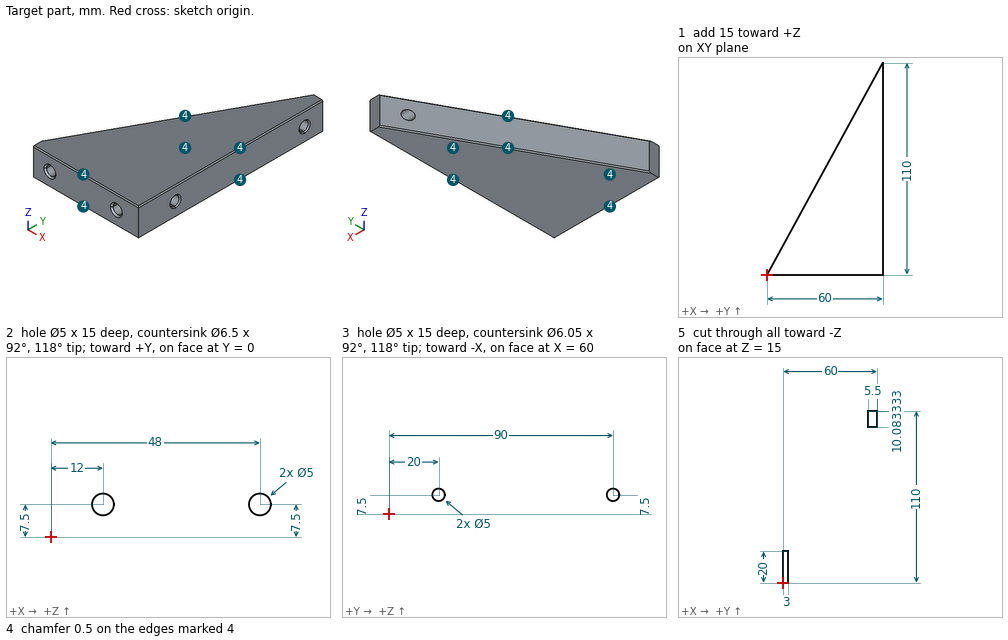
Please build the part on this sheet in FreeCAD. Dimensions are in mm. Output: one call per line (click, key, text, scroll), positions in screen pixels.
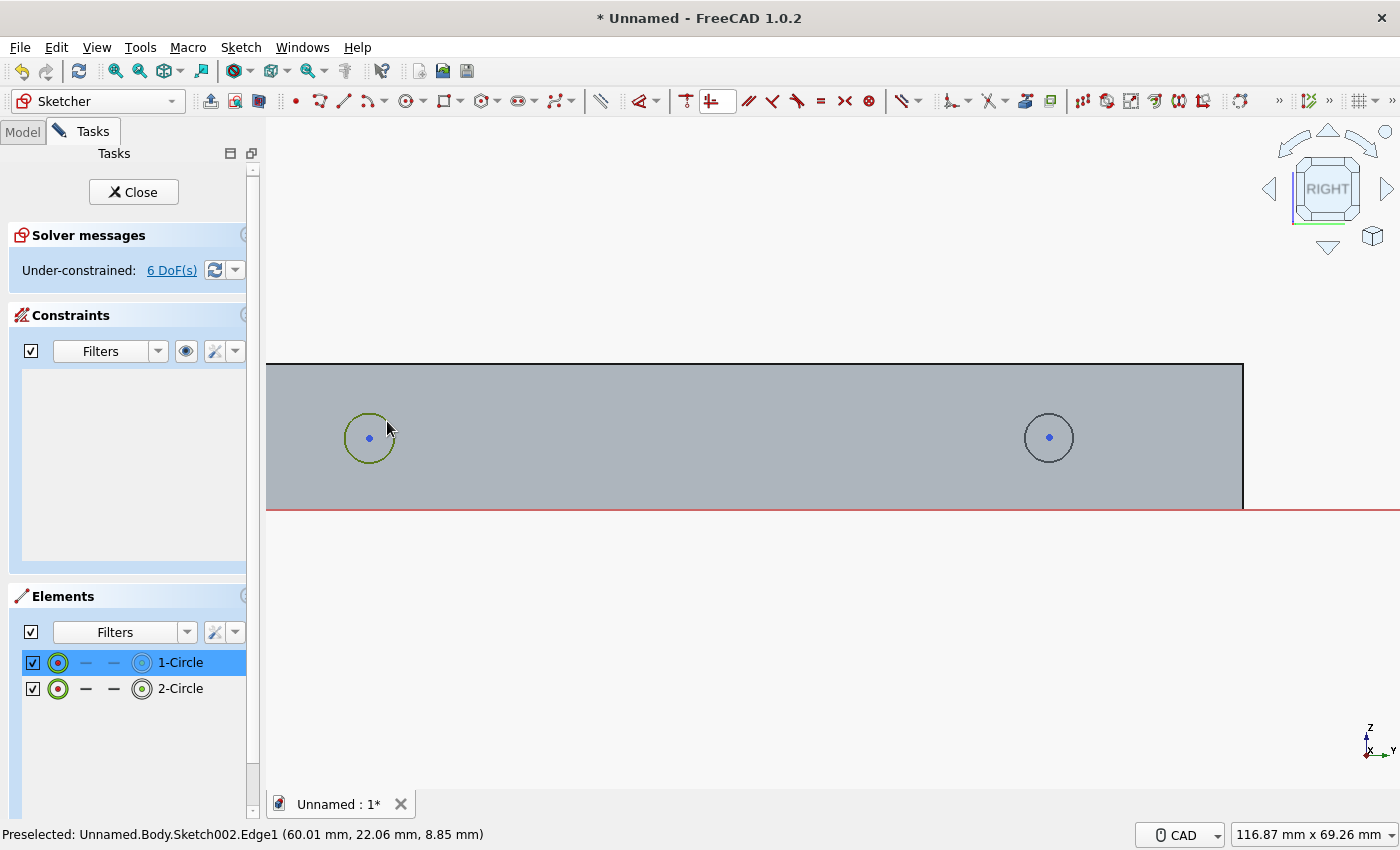
click(1066, 421)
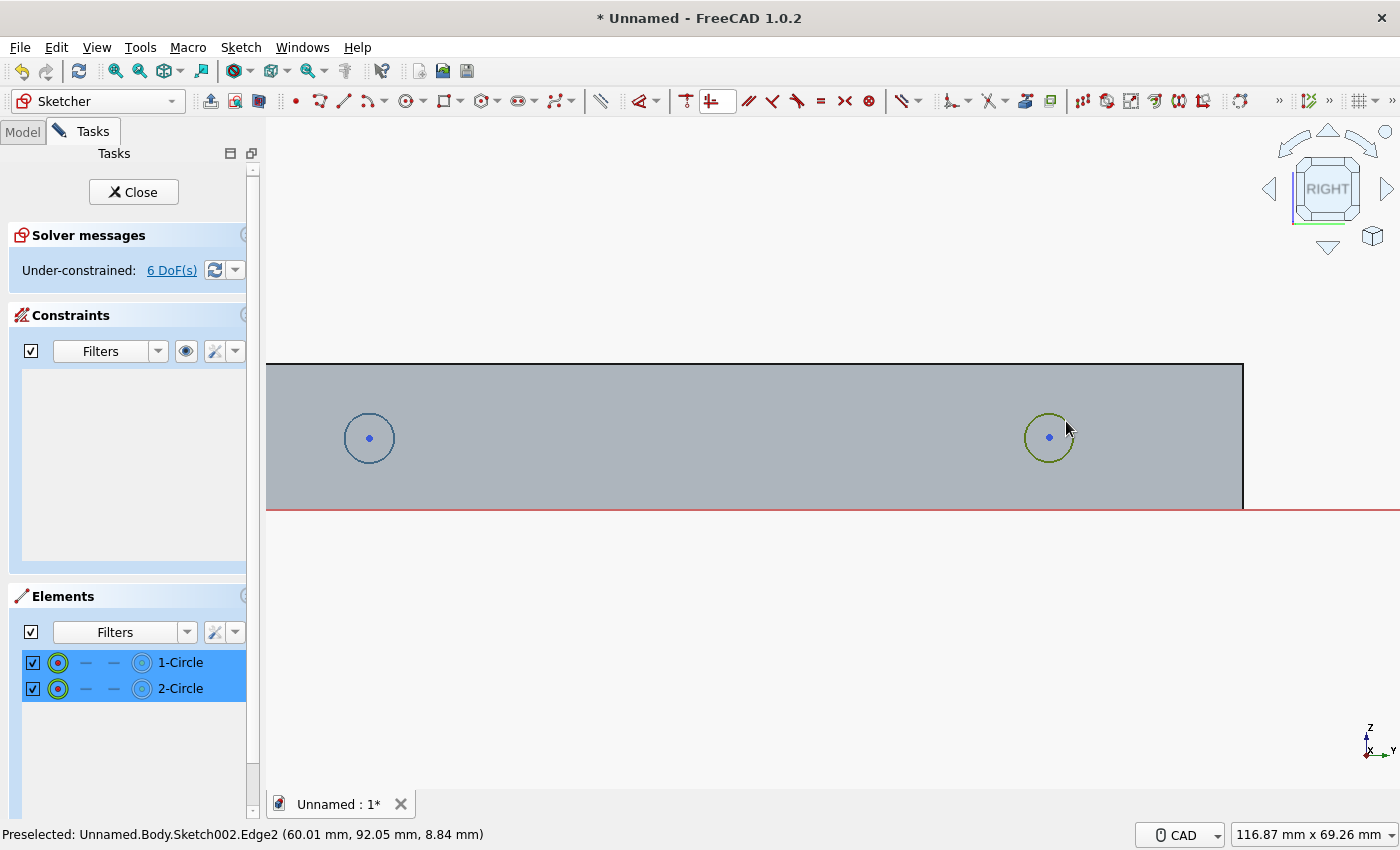
click(822, 102)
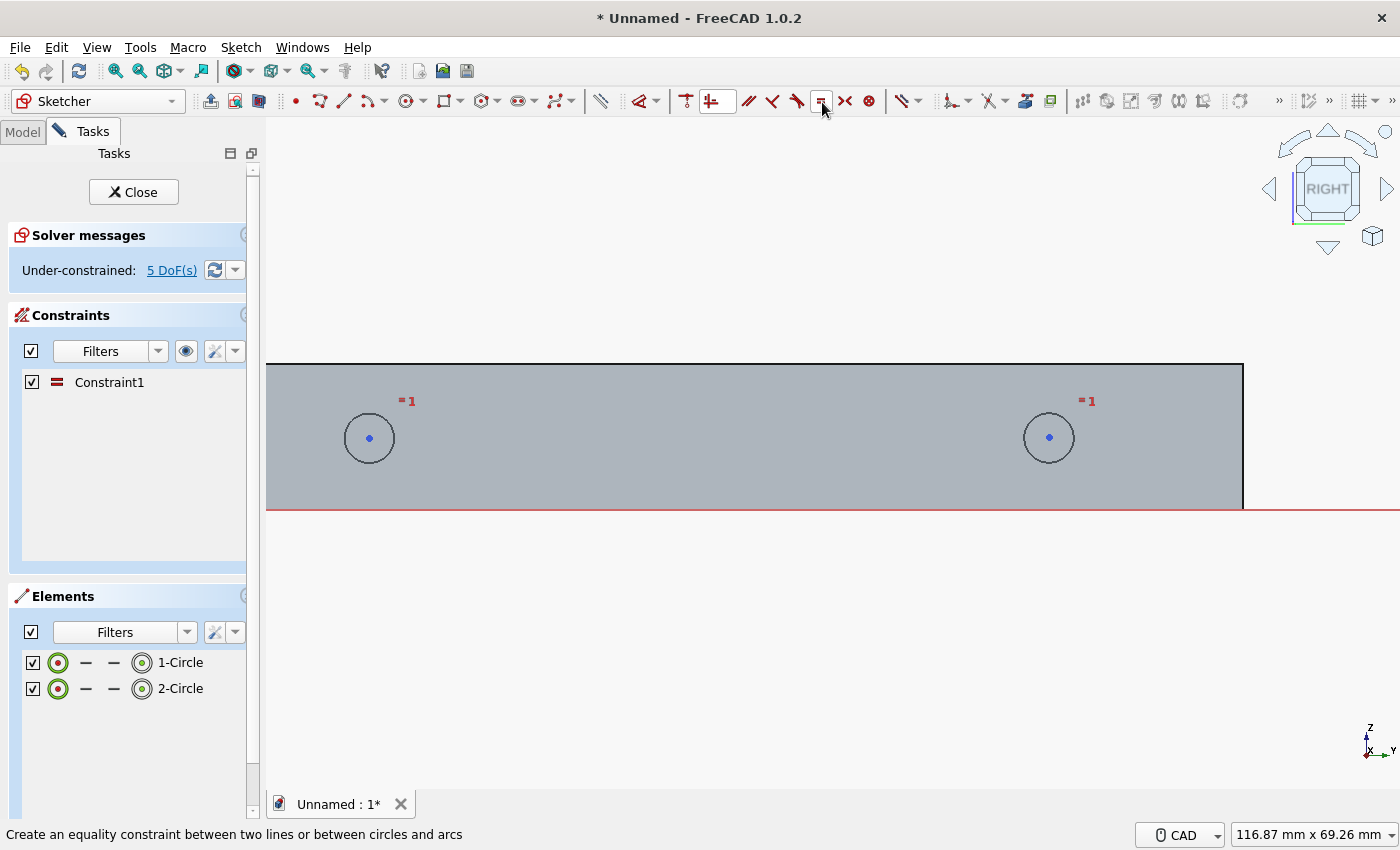
click(640, 102)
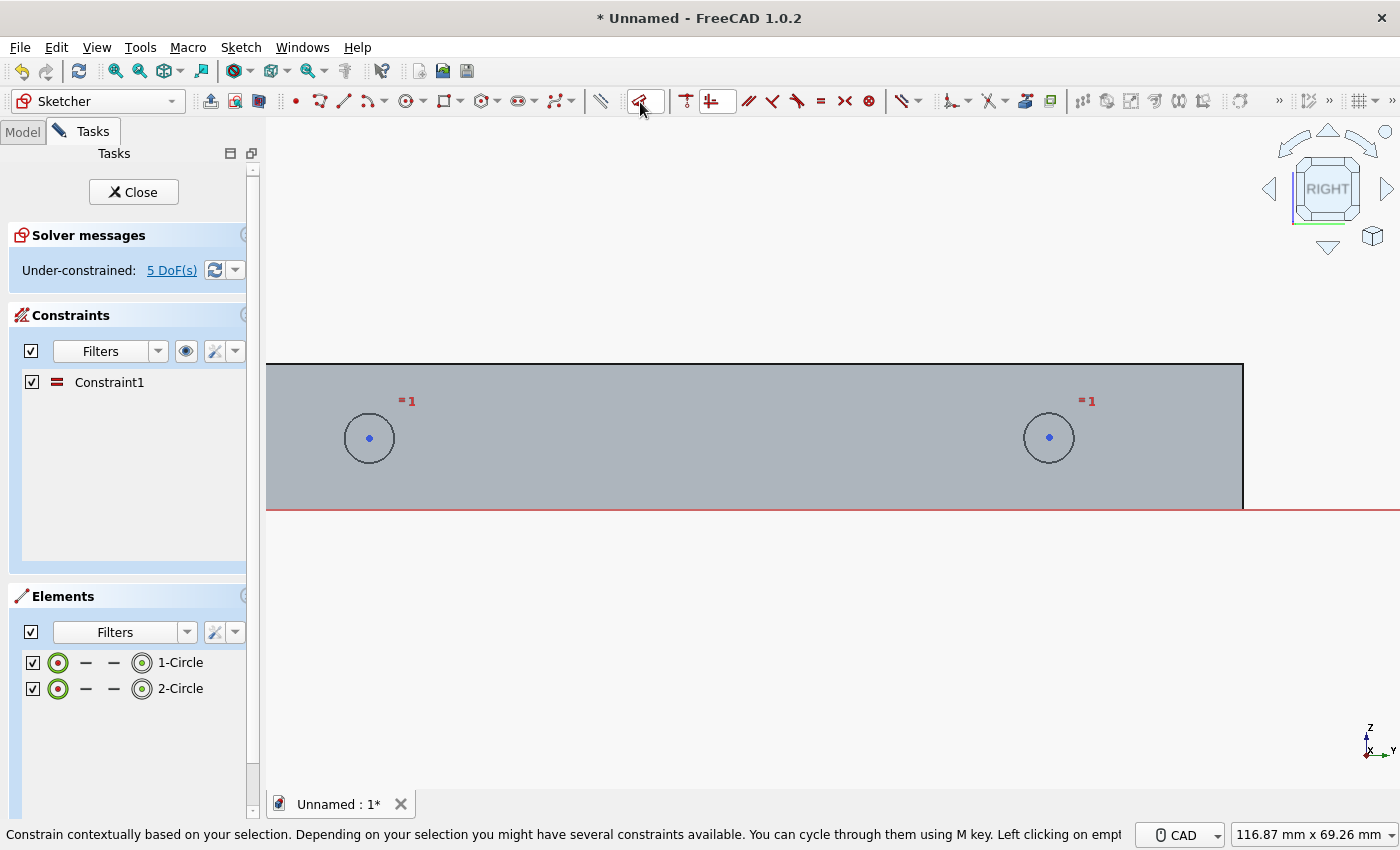
click(387, 421)
click(410, 399)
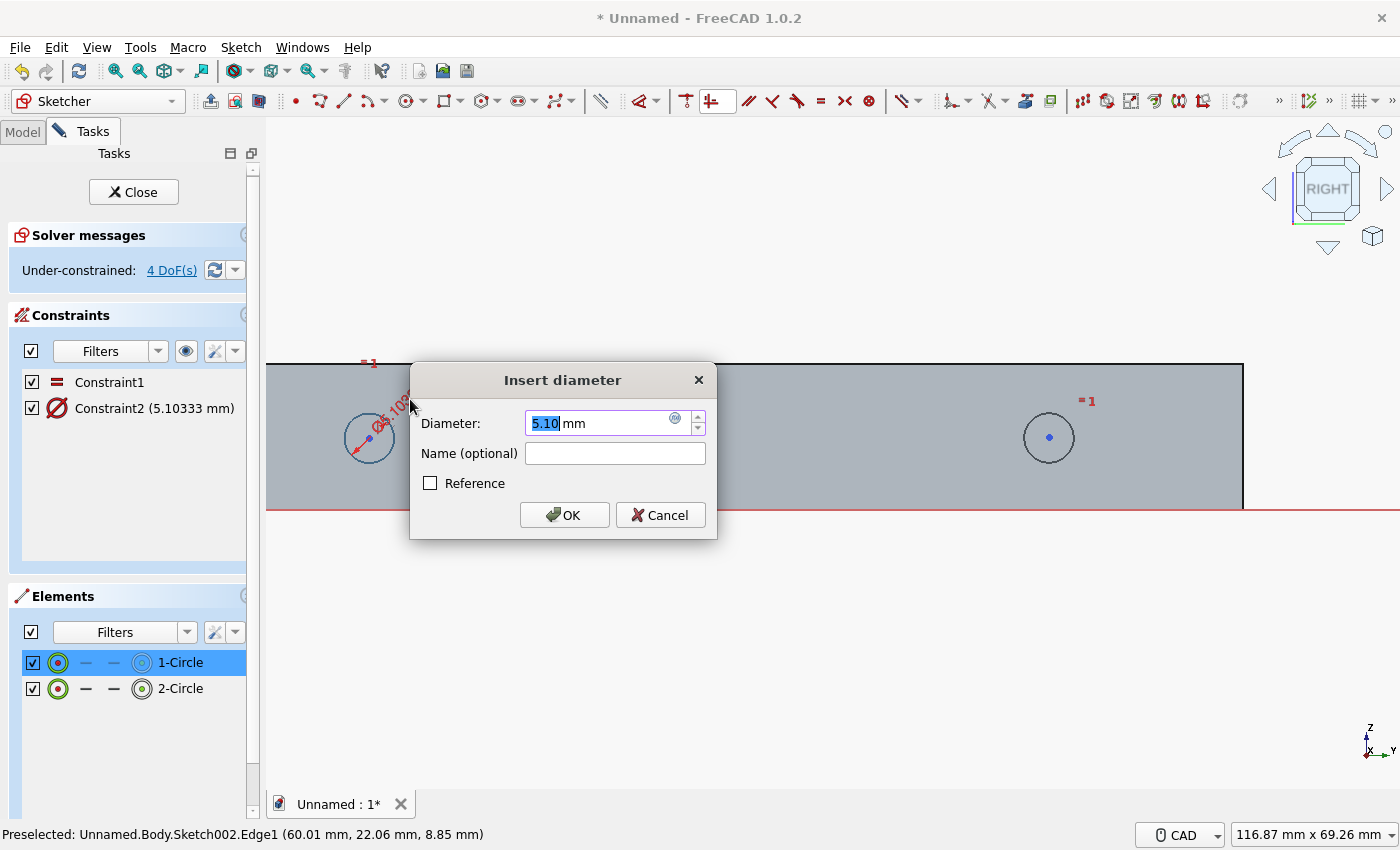
text(5)
key(Return)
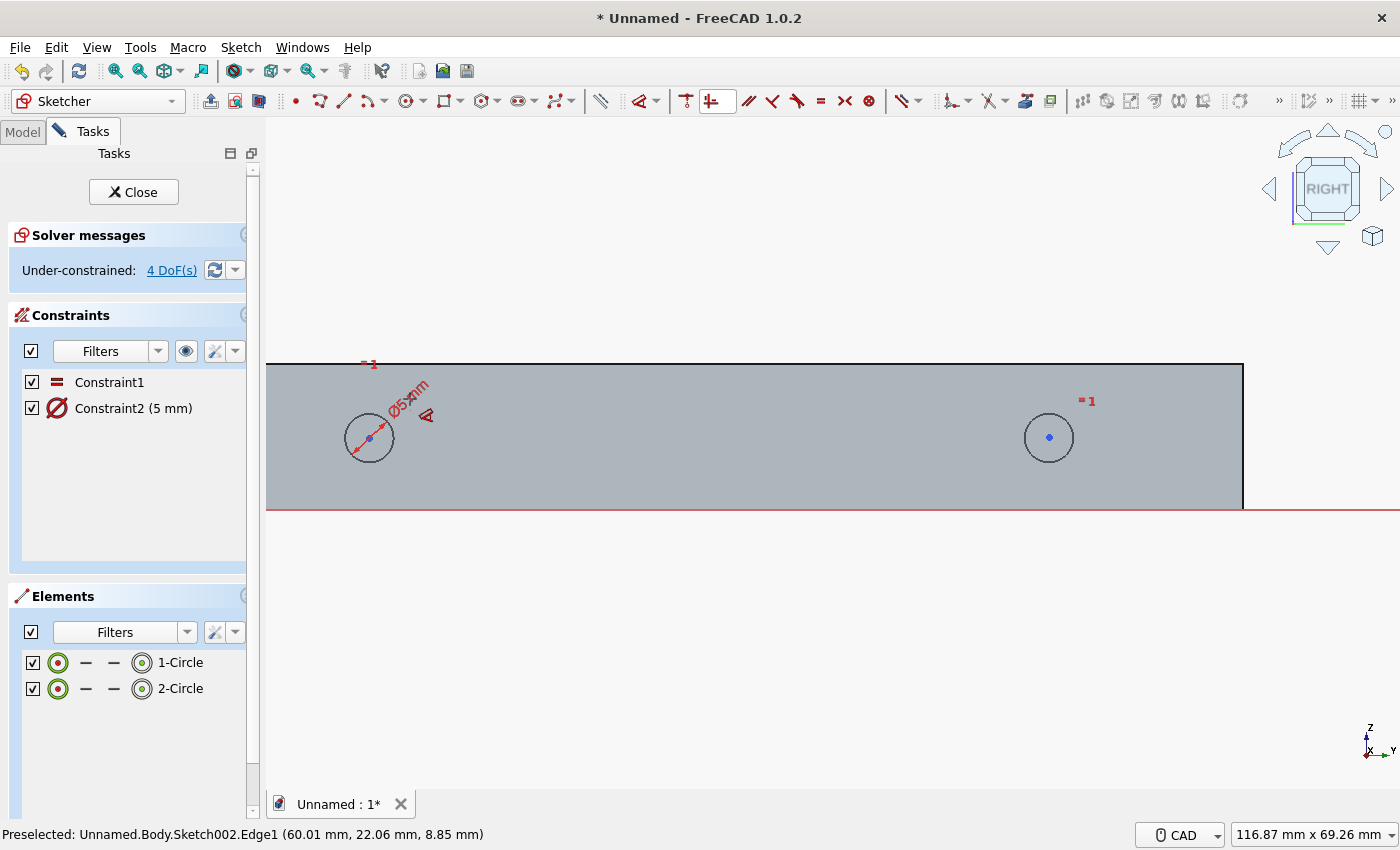
click(369, 438)
click(332, 544)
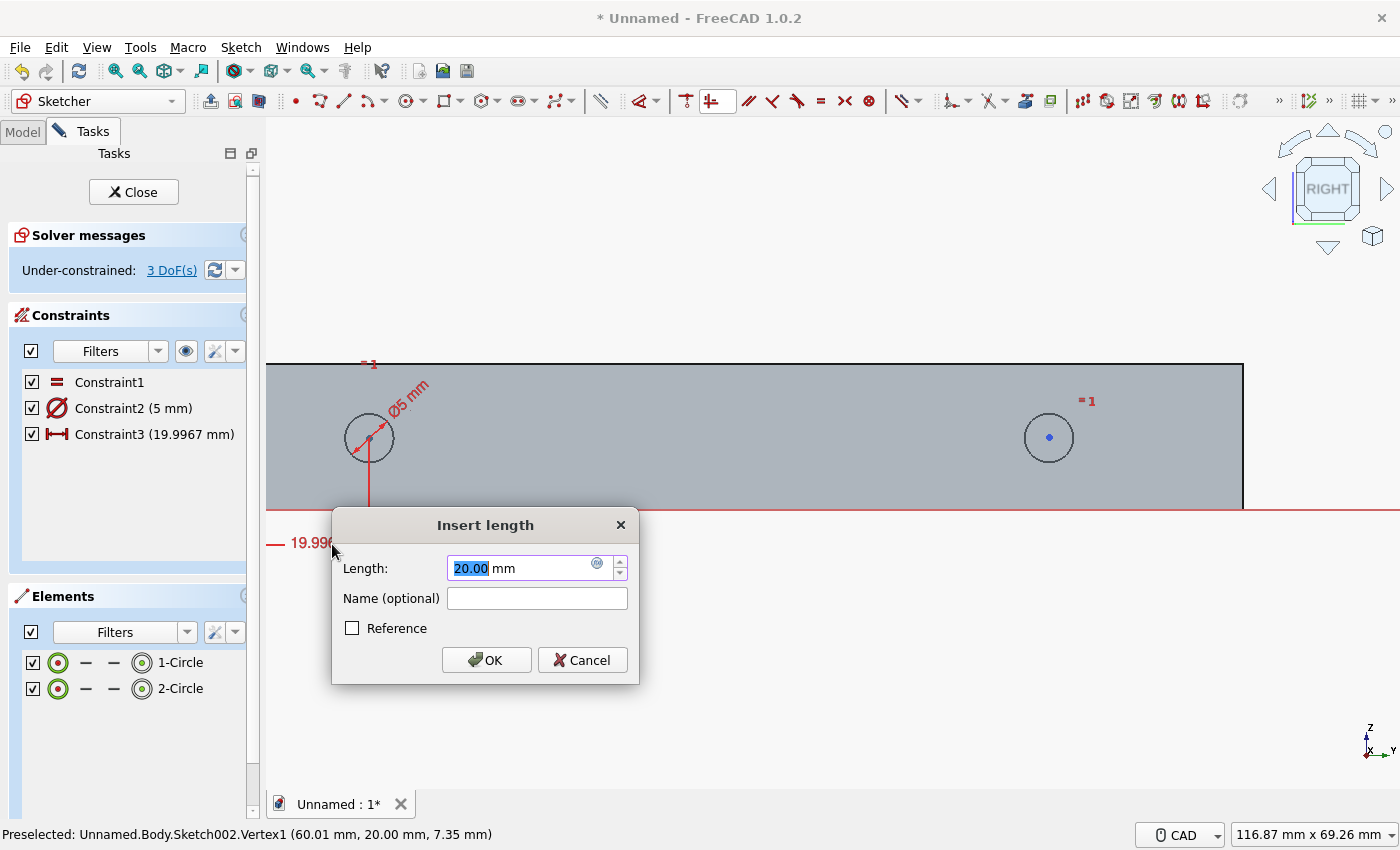
text(20)
key(Return)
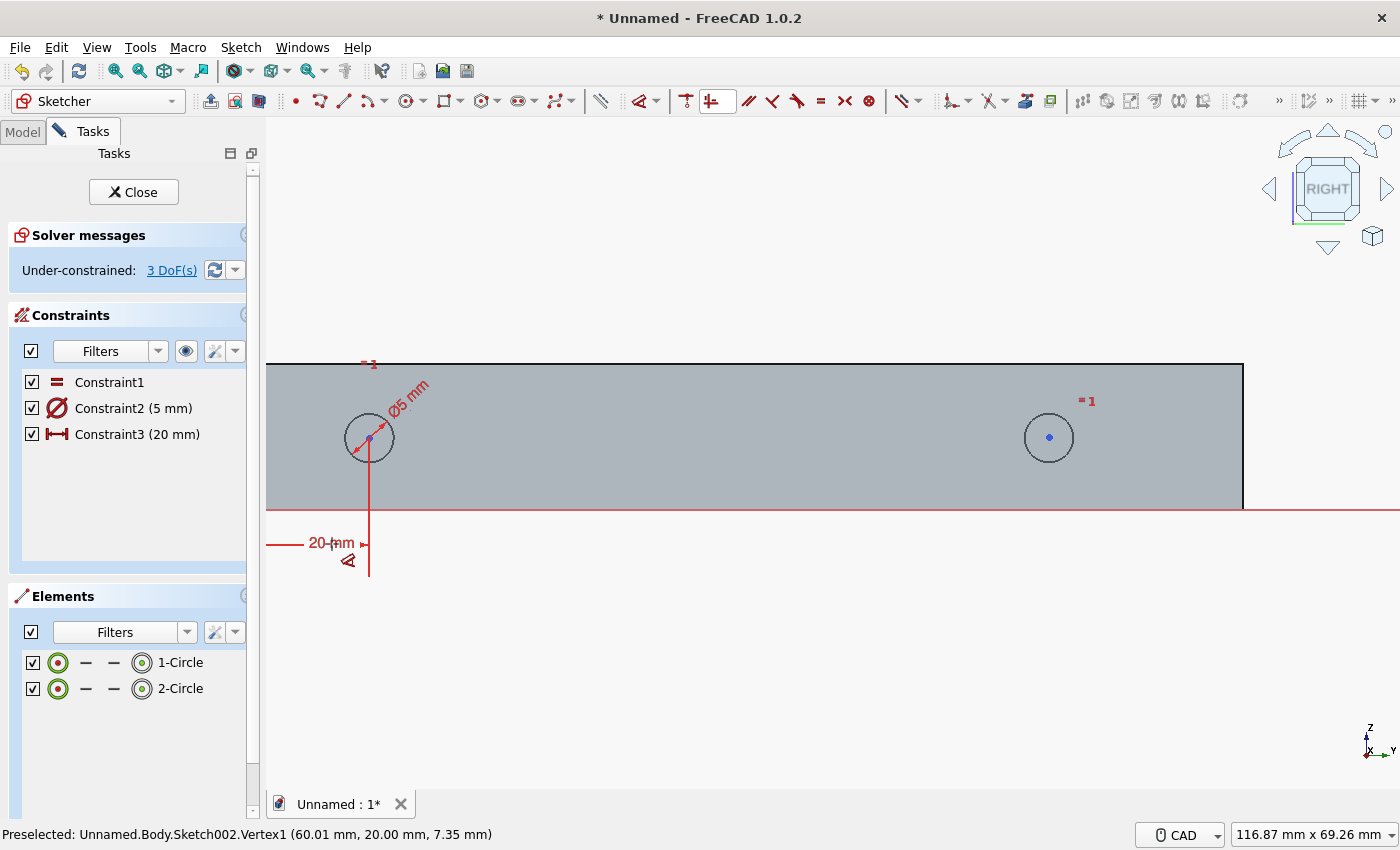
click(1049, 438)
click(671, 544)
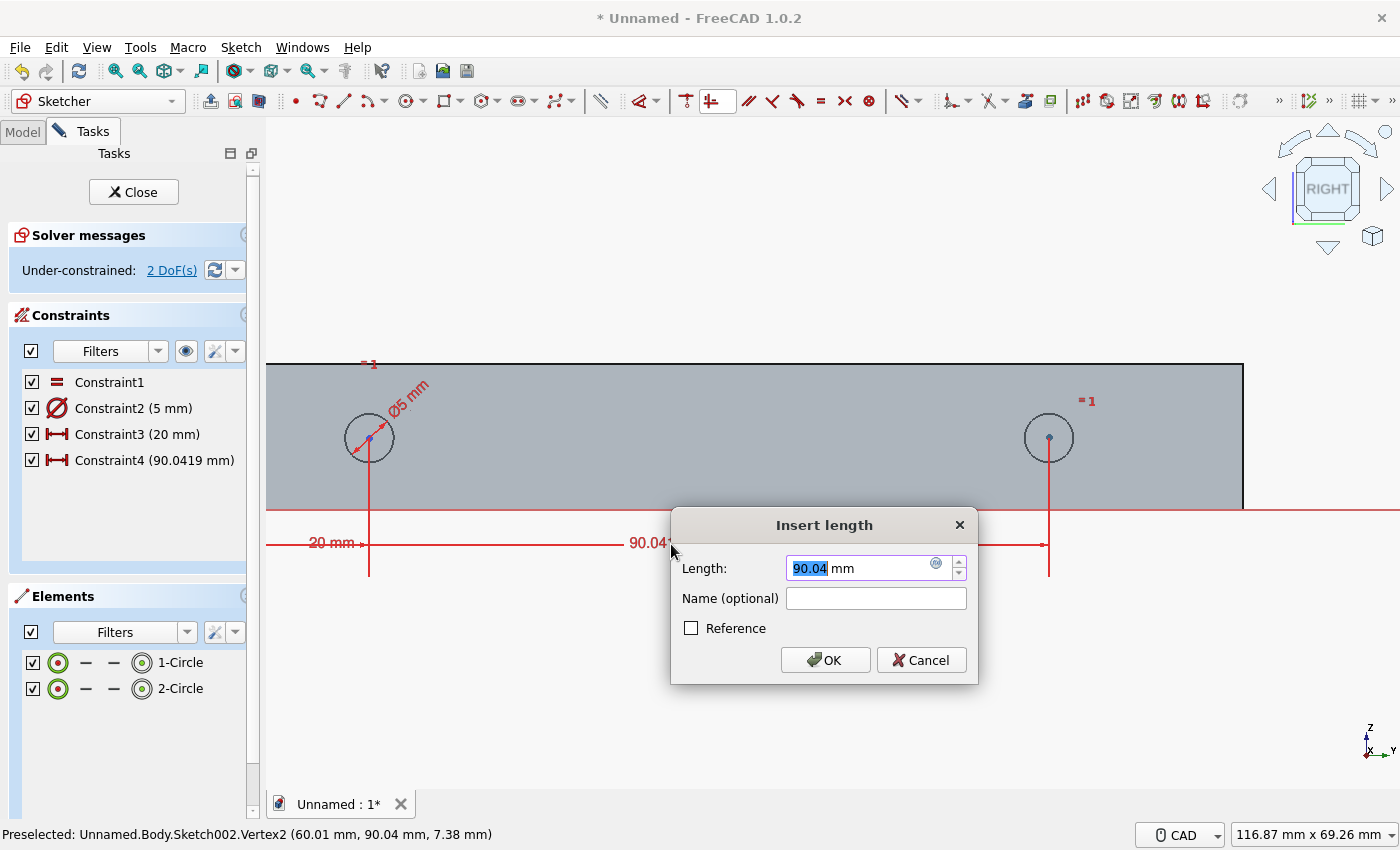
text(90)
key(Return)